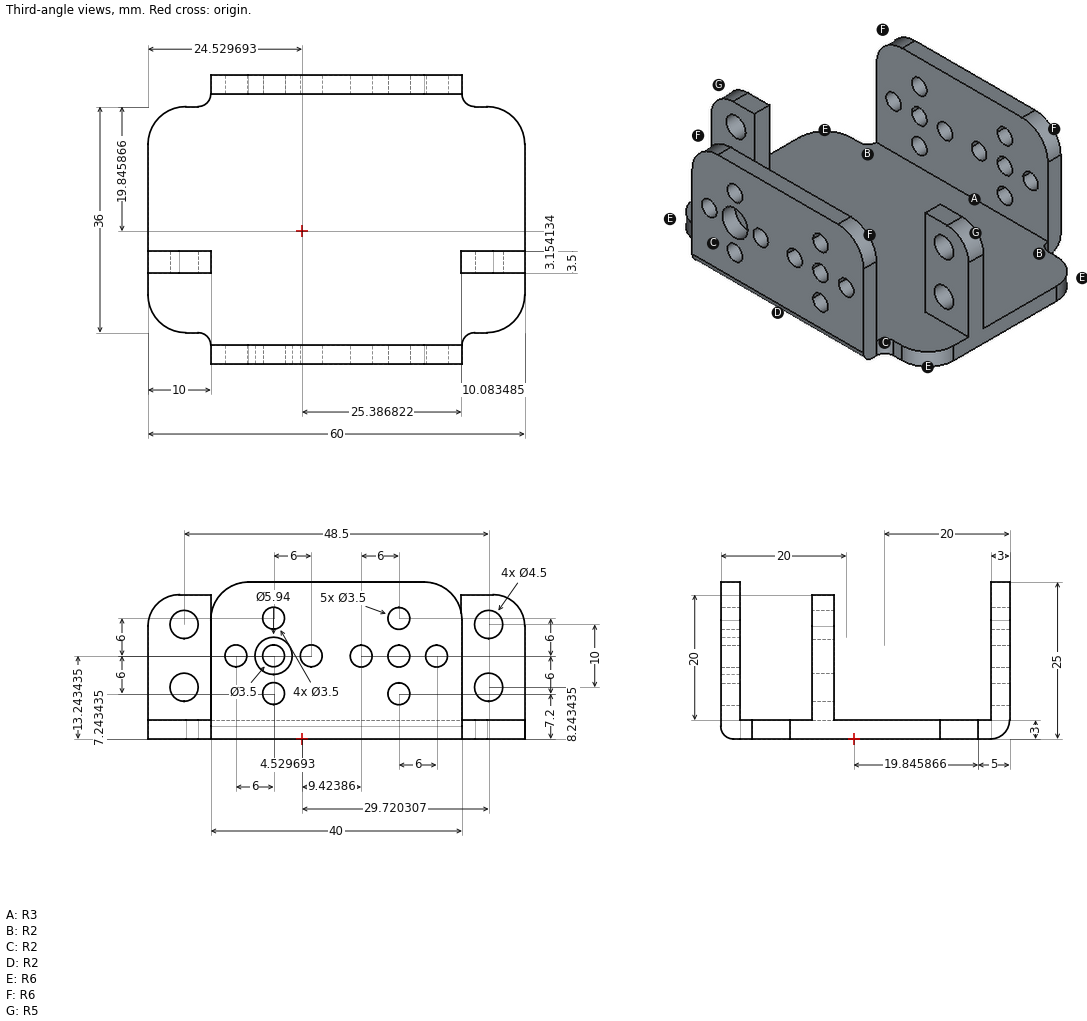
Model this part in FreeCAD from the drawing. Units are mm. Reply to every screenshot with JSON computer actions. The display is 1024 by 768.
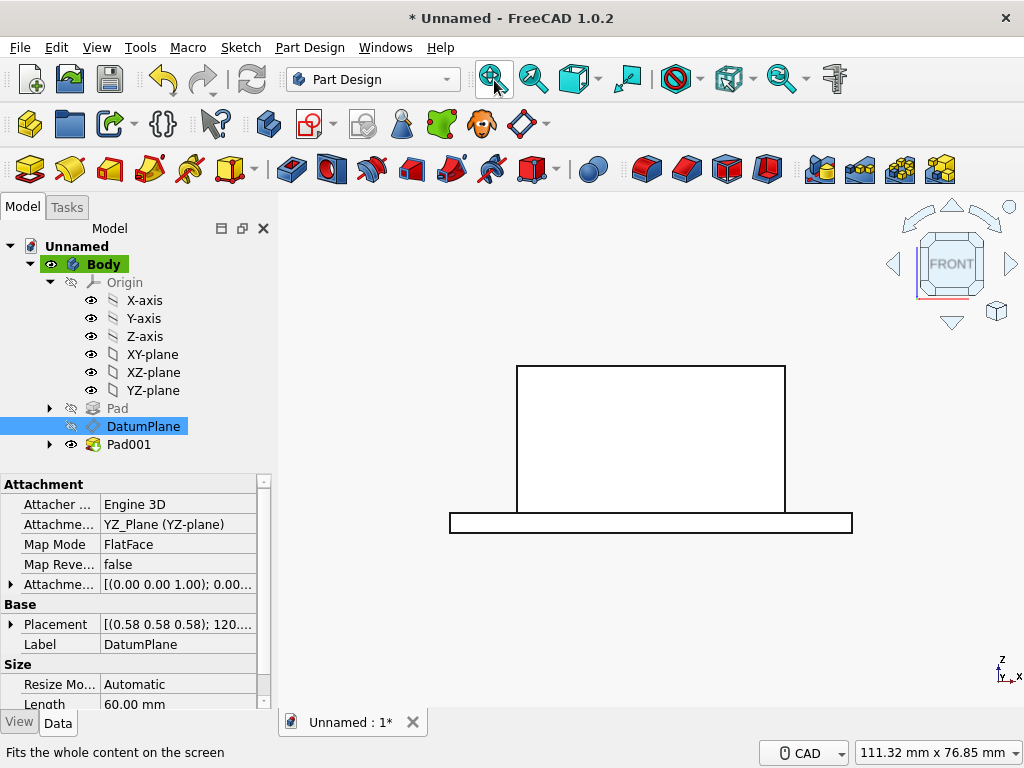
{"action": "key", "text": "3"}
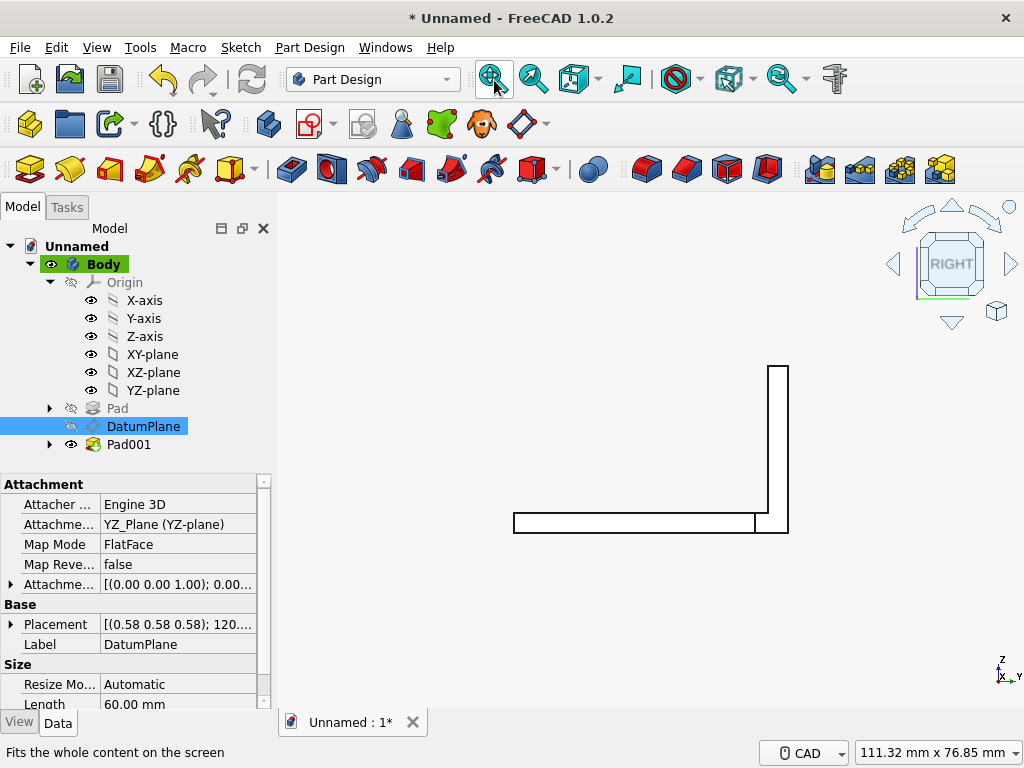
{"action": "left_click", "coordinate": [494, 80]}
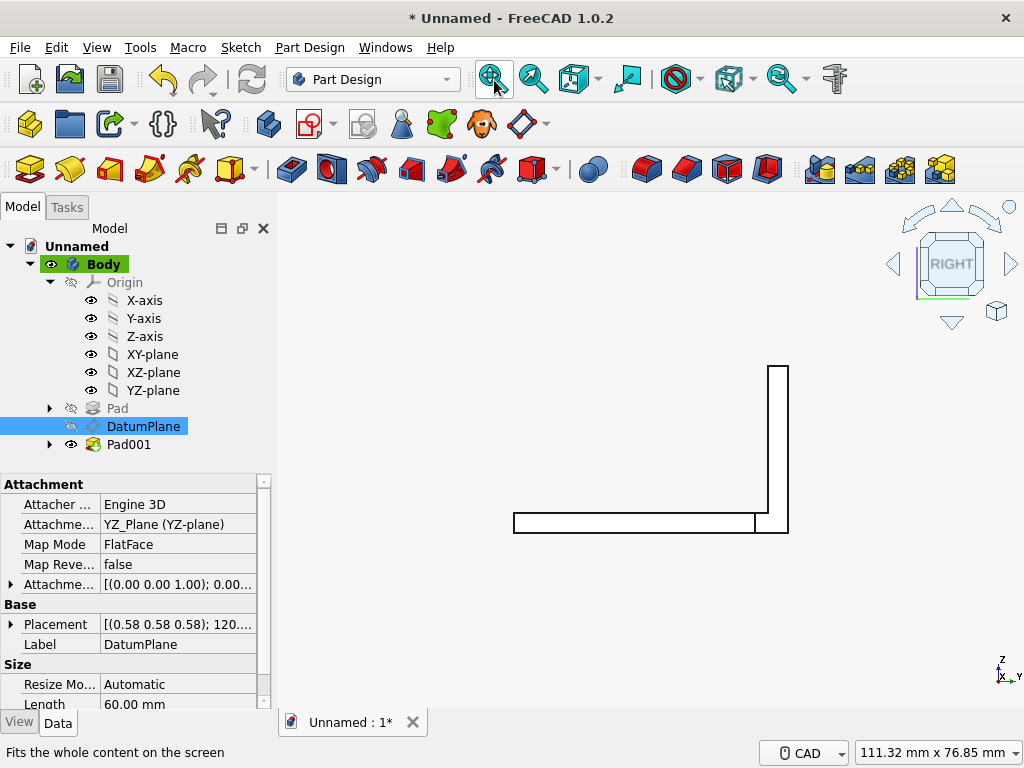
{"action": "key", "text": "5"}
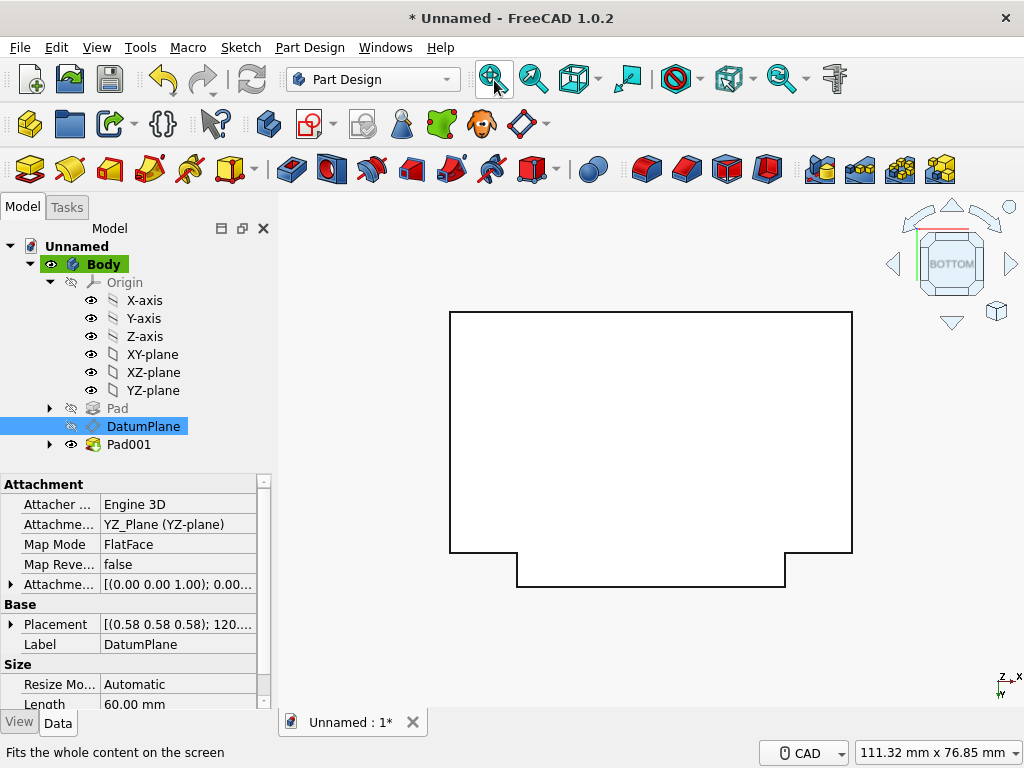
{"action": "left_click", "coordinate": [651, 586]}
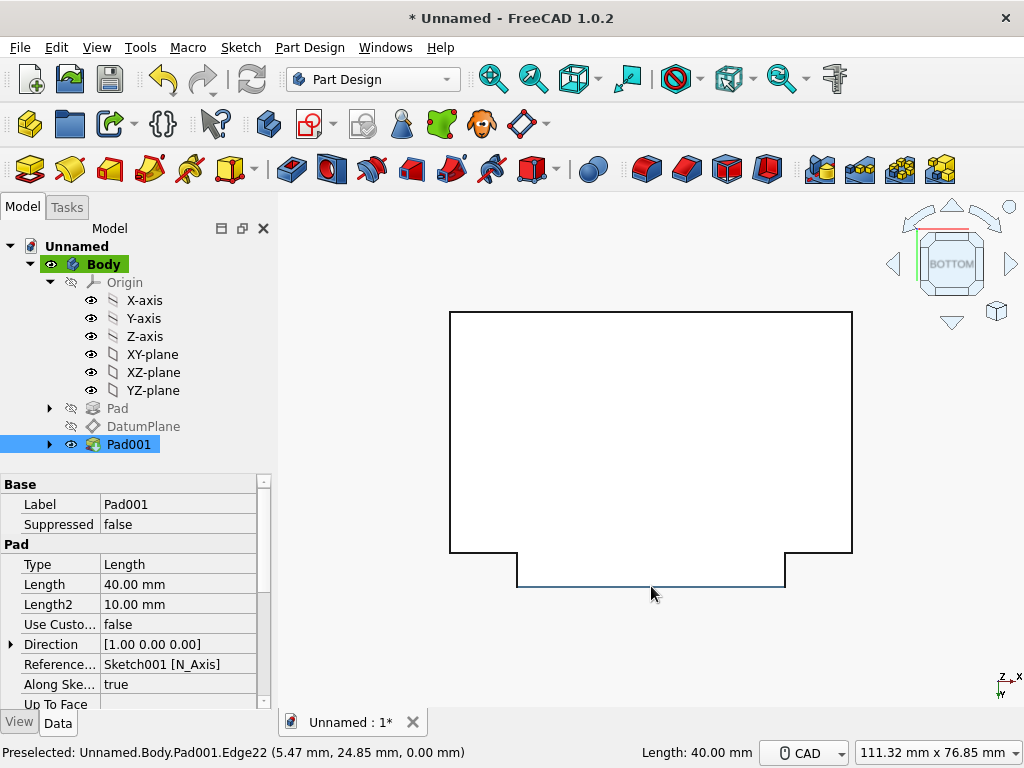
{"action": "left_click", "coordinate": [648, 170]}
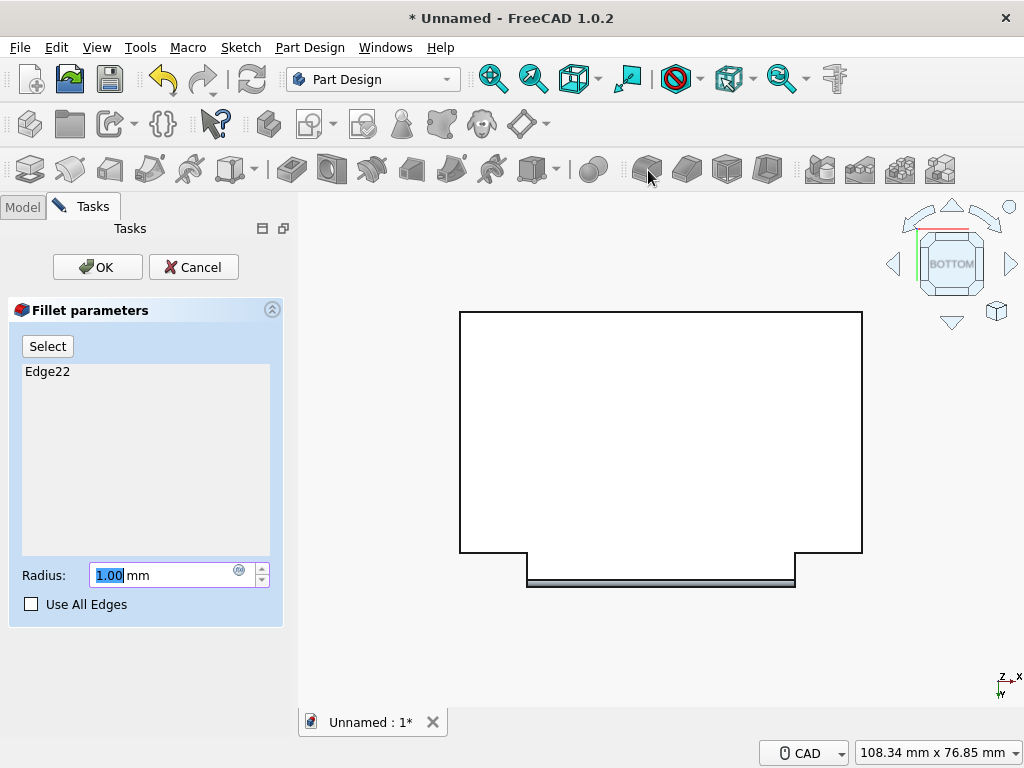
{"action": "type", "text": "3"}
{"action": "key", "text": "Tab"}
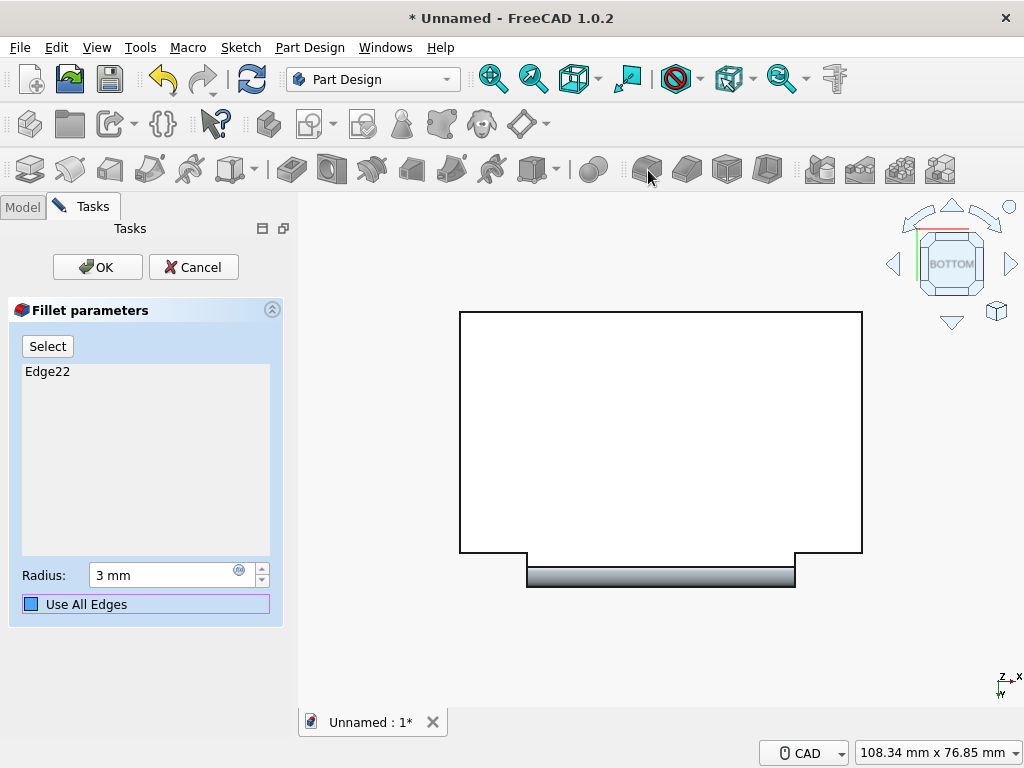
{"action": "left_click", "coordinate": [98, 267]}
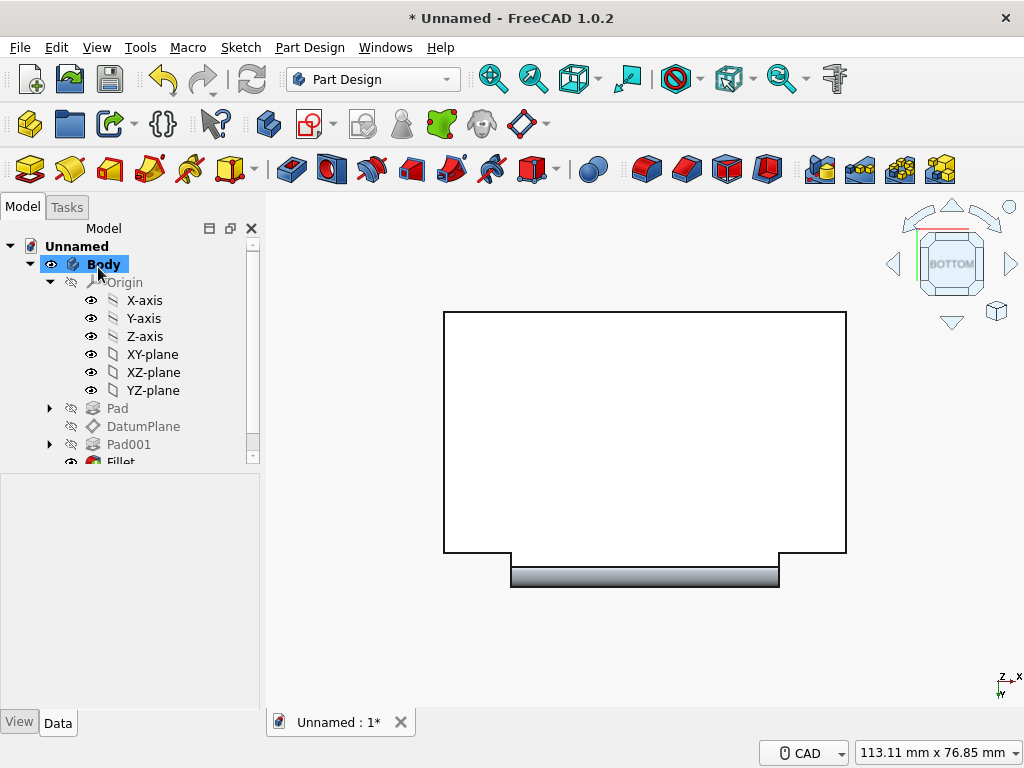
{"action": "scroll", "coordinate": [511, 552], "scroll_direction": "up", "scroll_amount": 4}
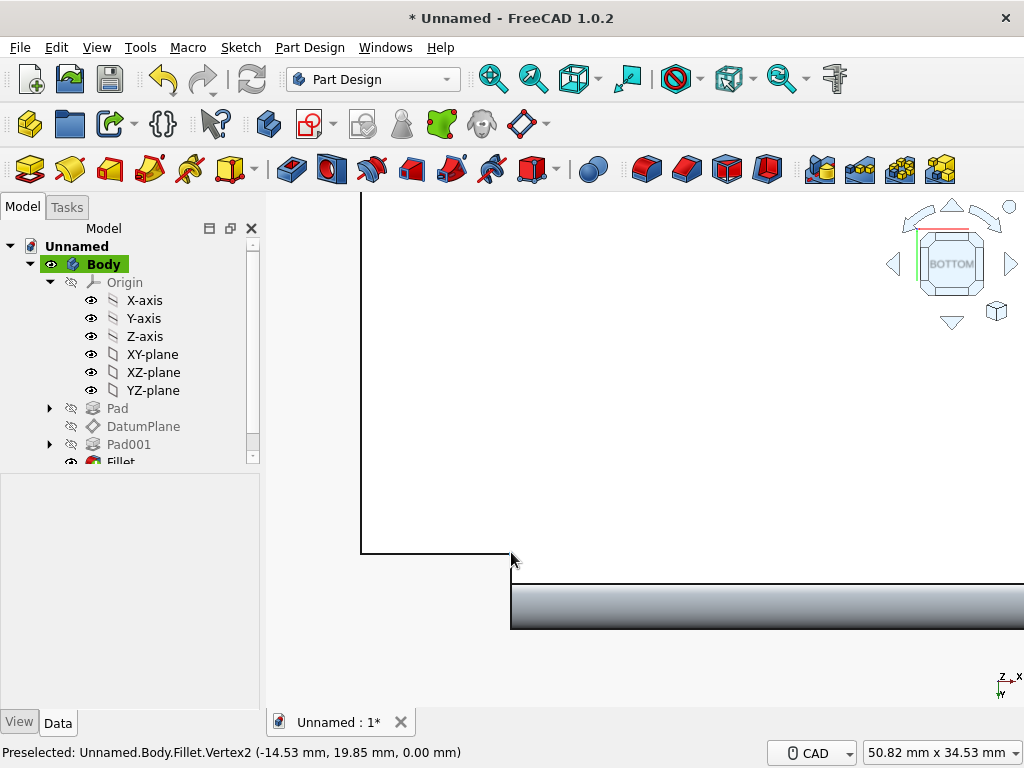
{"action": "left_click", "coordinate": [494, 80]}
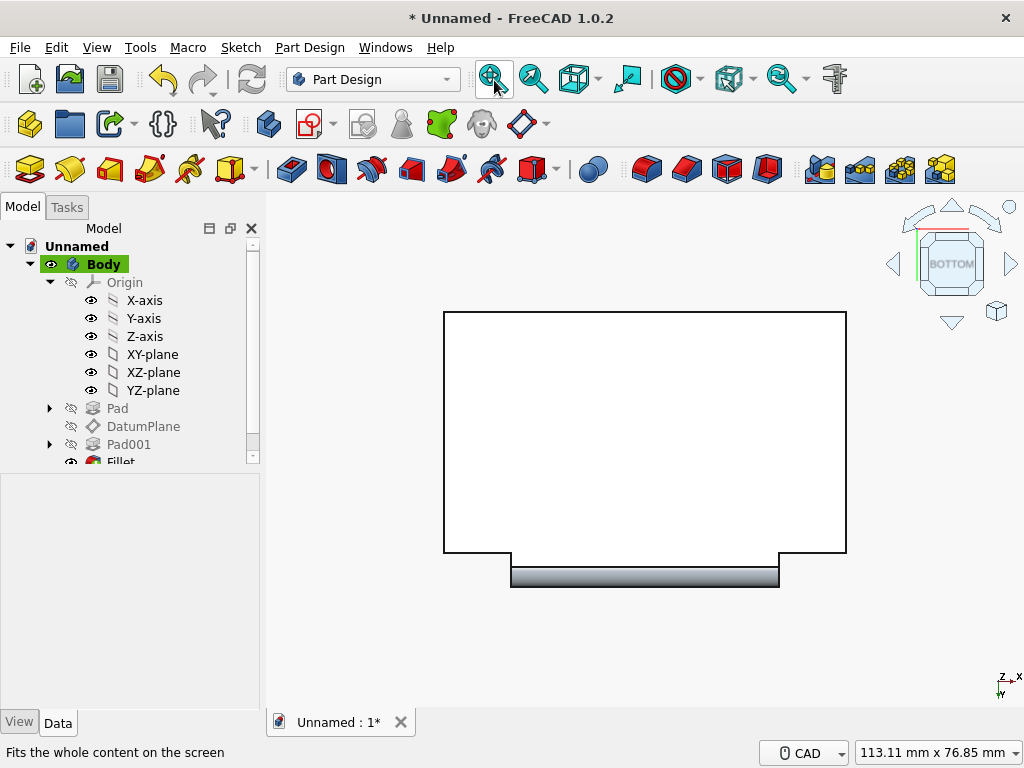
{"action": "key", "text": "0"}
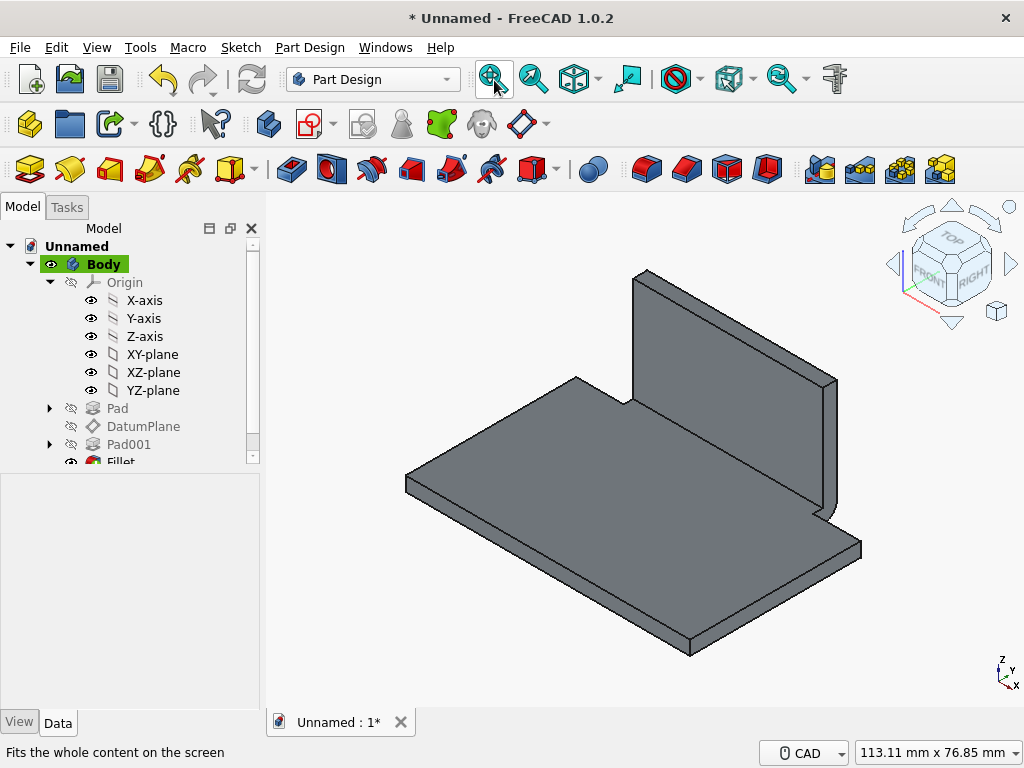
{"action": "scroll", "coordinate": [624, 412], "scroll_direction": "up", "scroll_amount": 4}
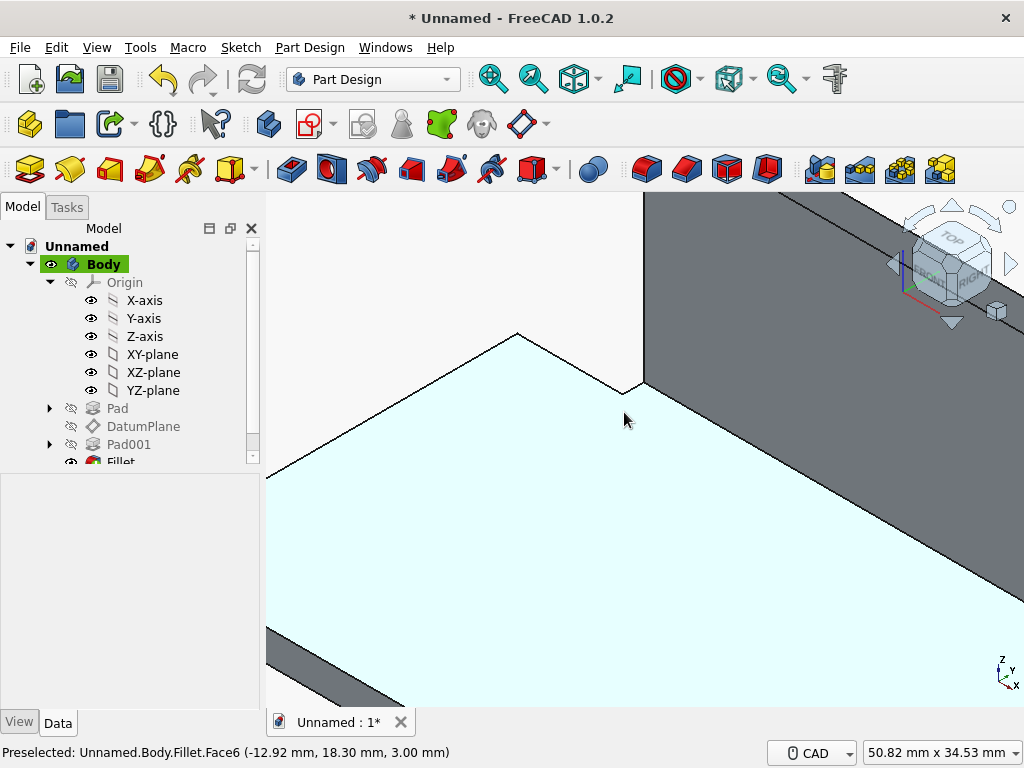
{"action": "left_click", "coordinate": [494, 80]}